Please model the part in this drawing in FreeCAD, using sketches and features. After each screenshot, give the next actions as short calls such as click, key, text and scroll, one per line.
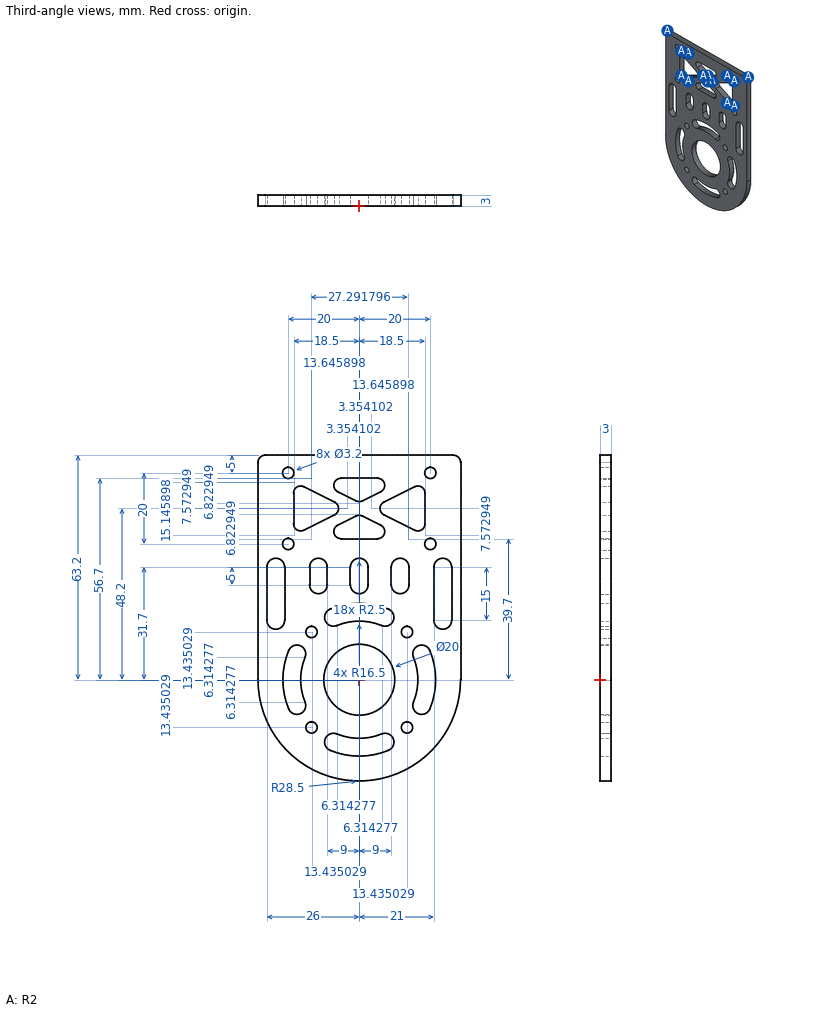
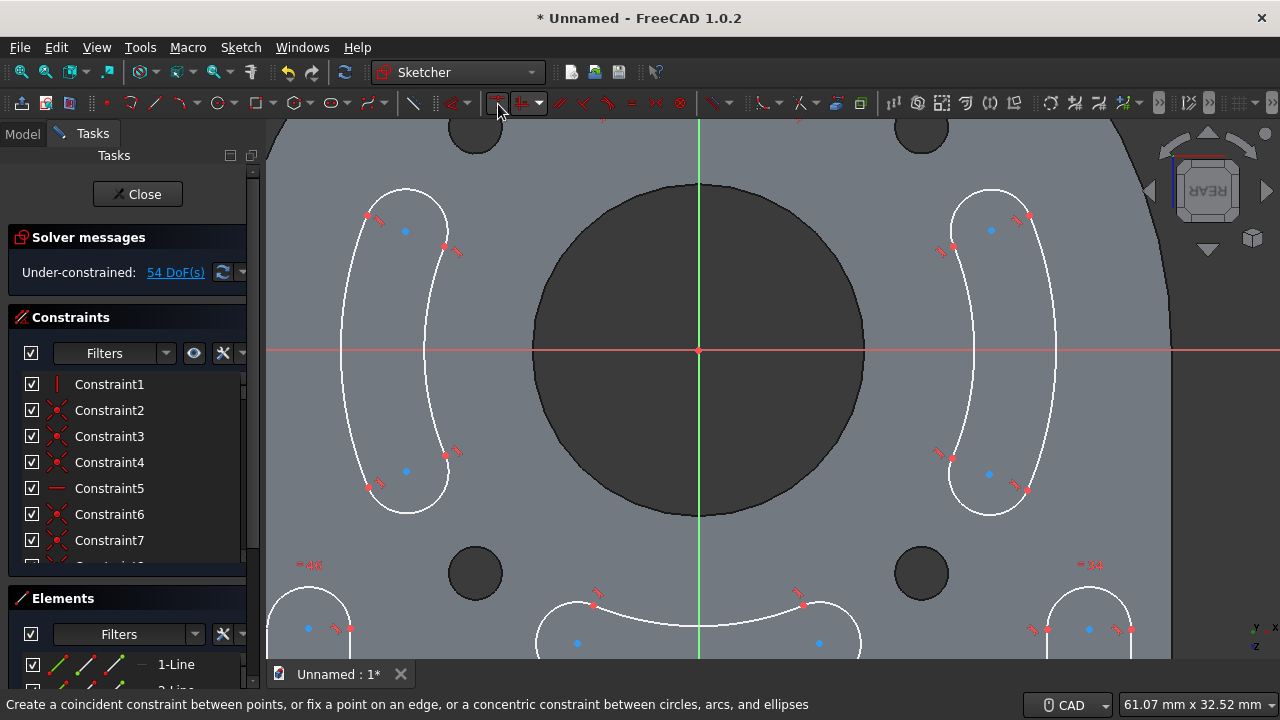
scroll(706, 306, down, 7)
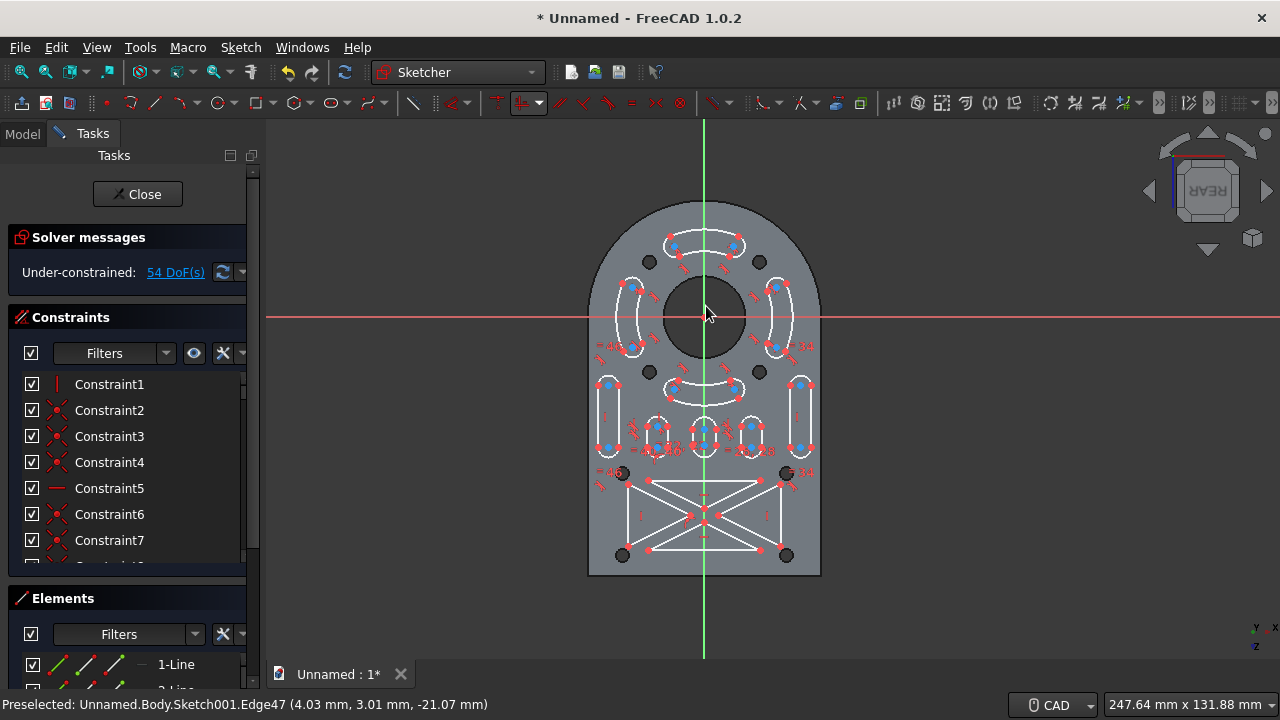
scroll(697, 455, up, 4)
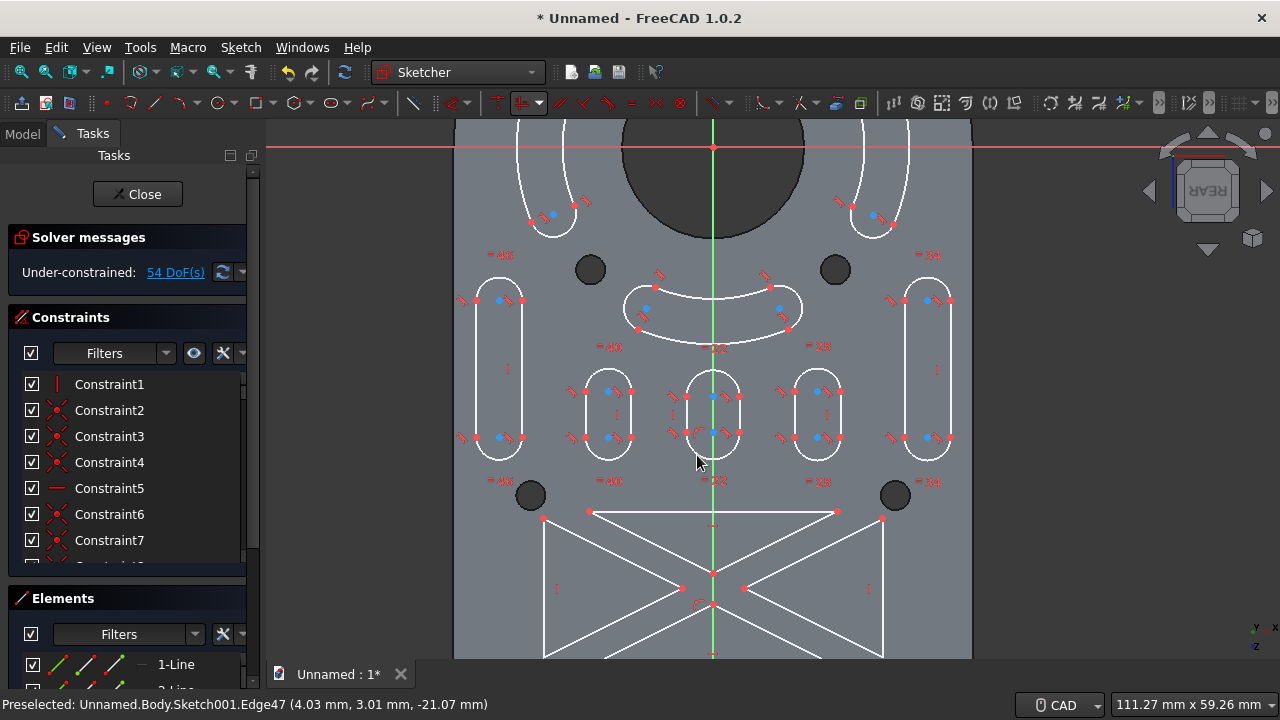
click(698, 454)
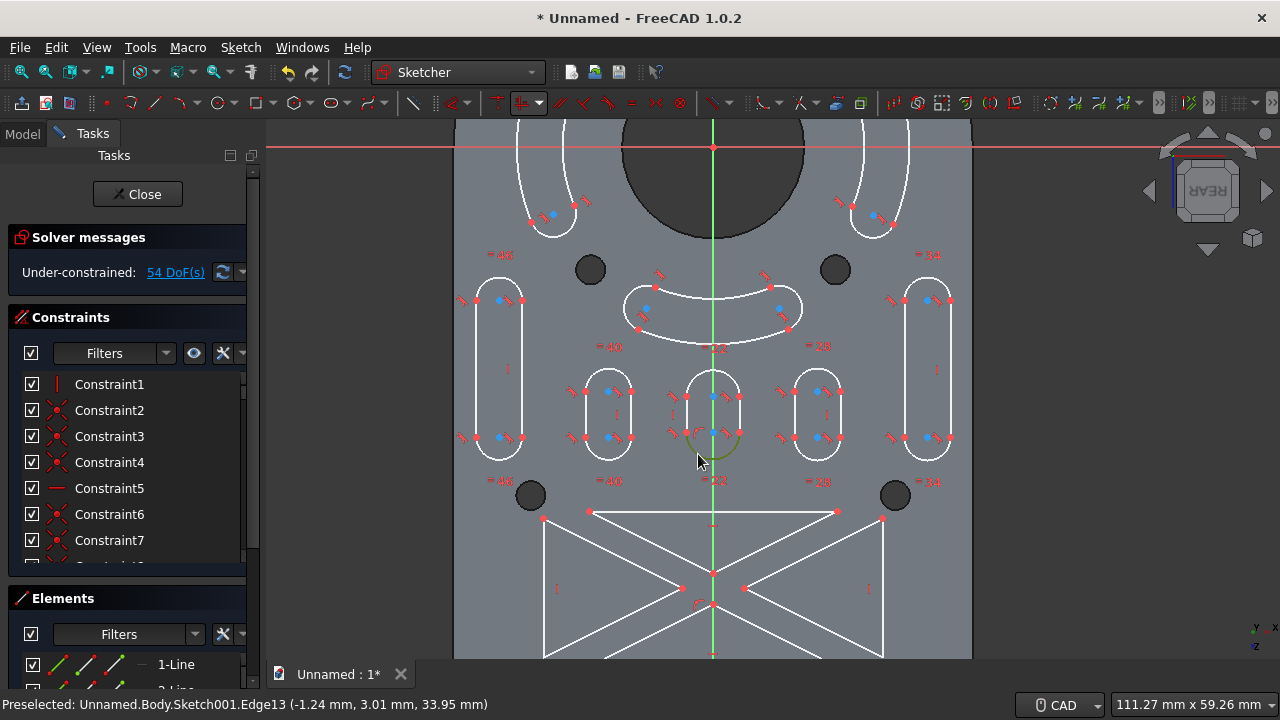
click(804, 456)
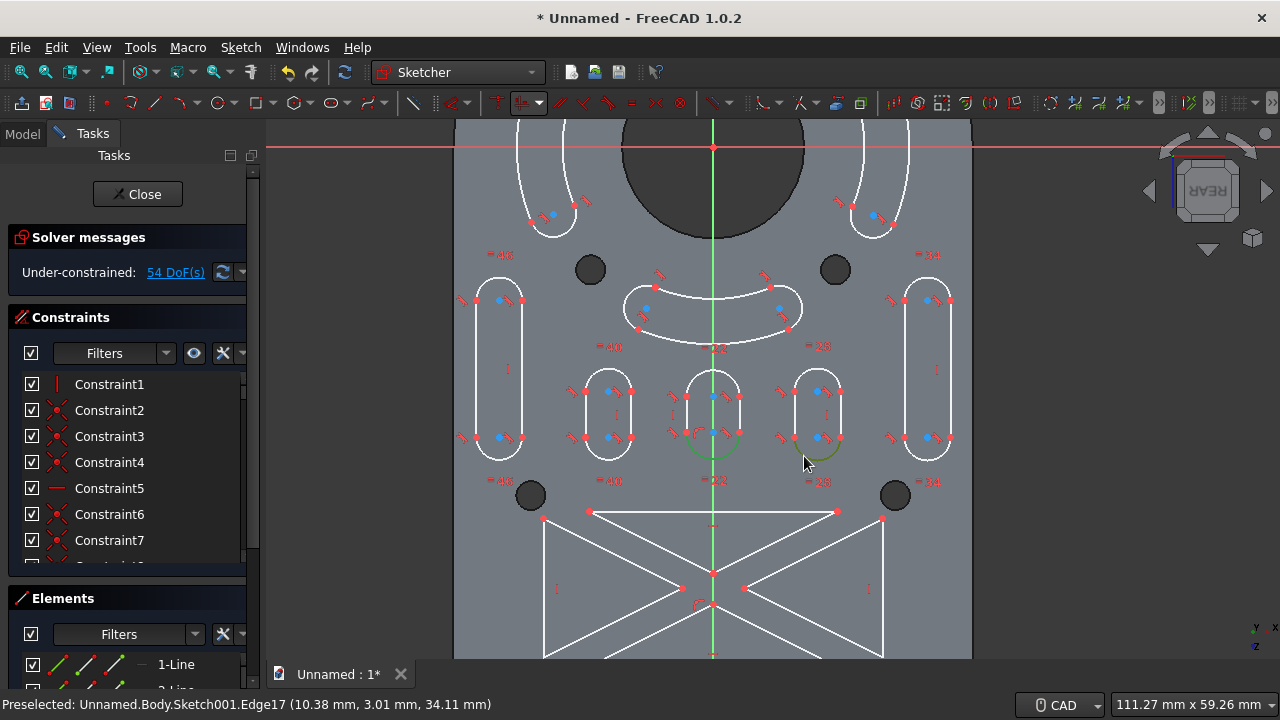
click(914, 456)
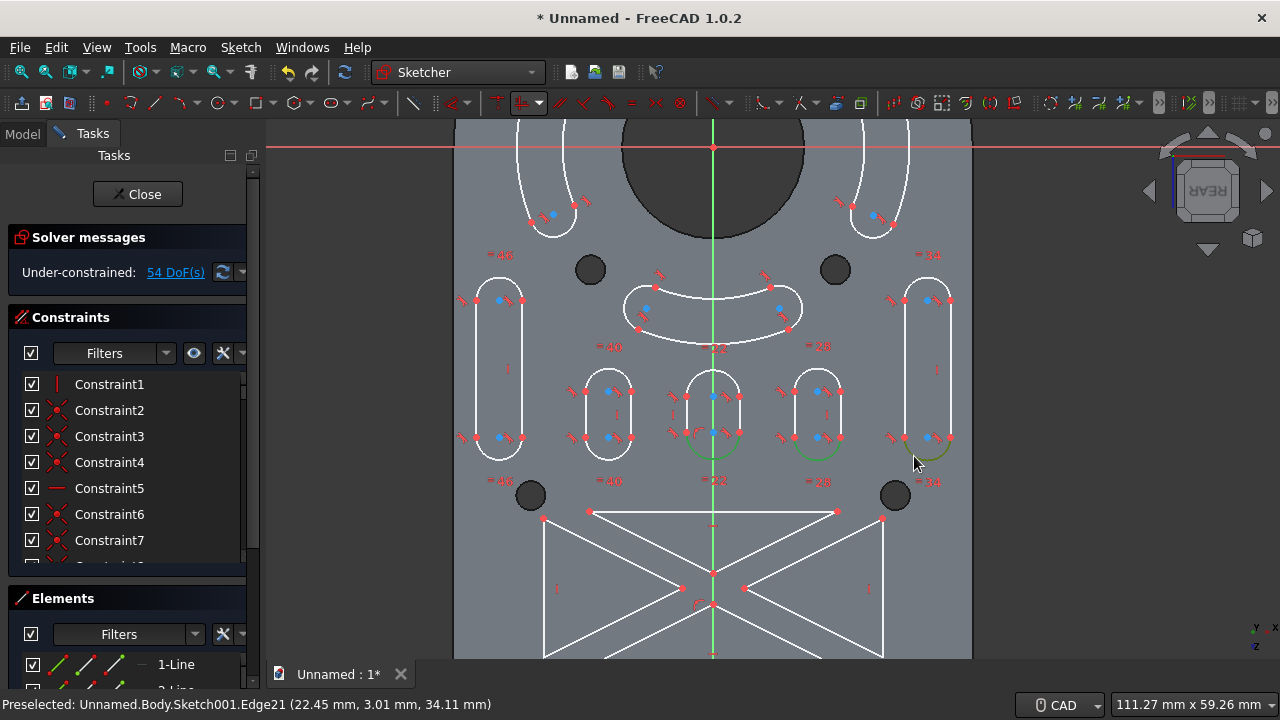
click(635, 289)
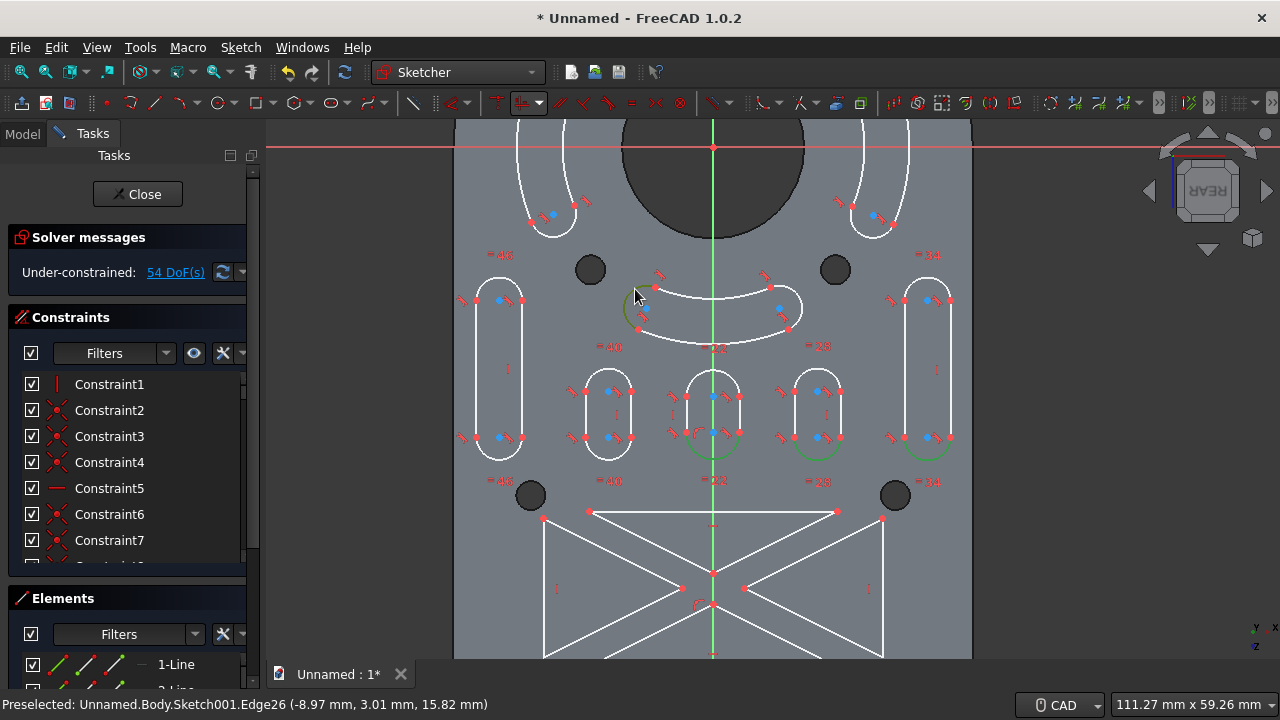
click(595, 455)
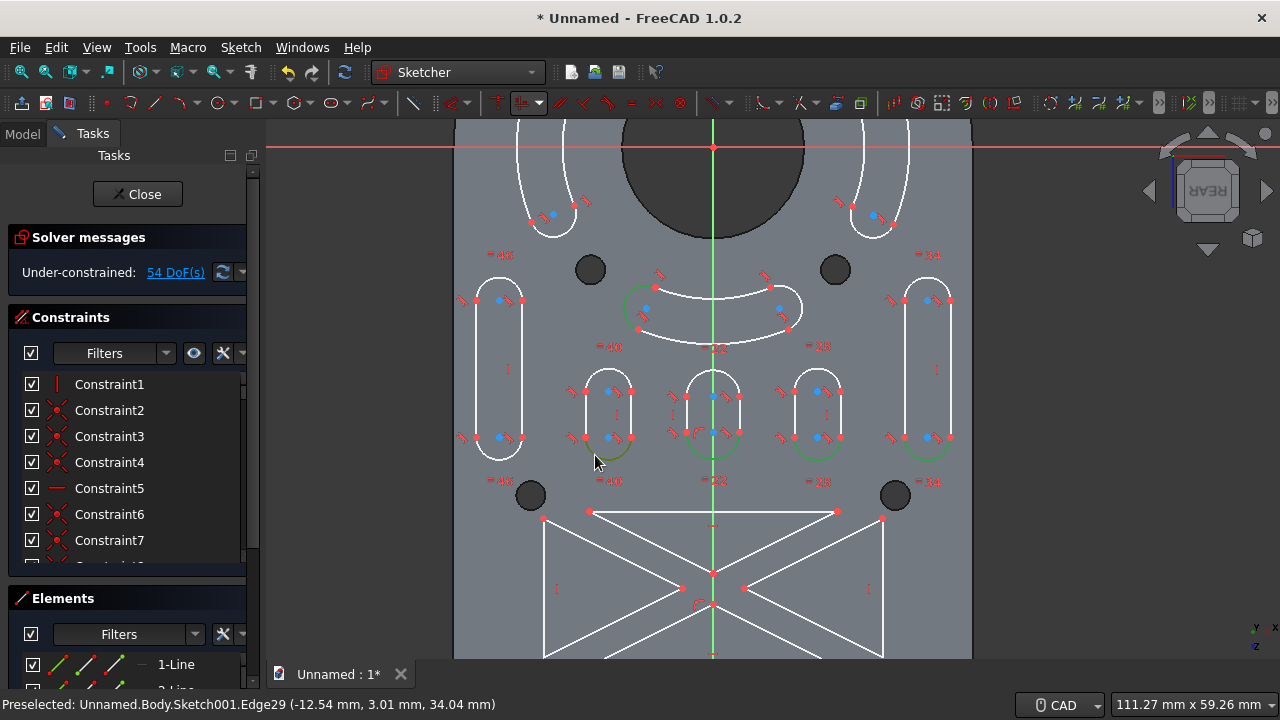
click(486, 455)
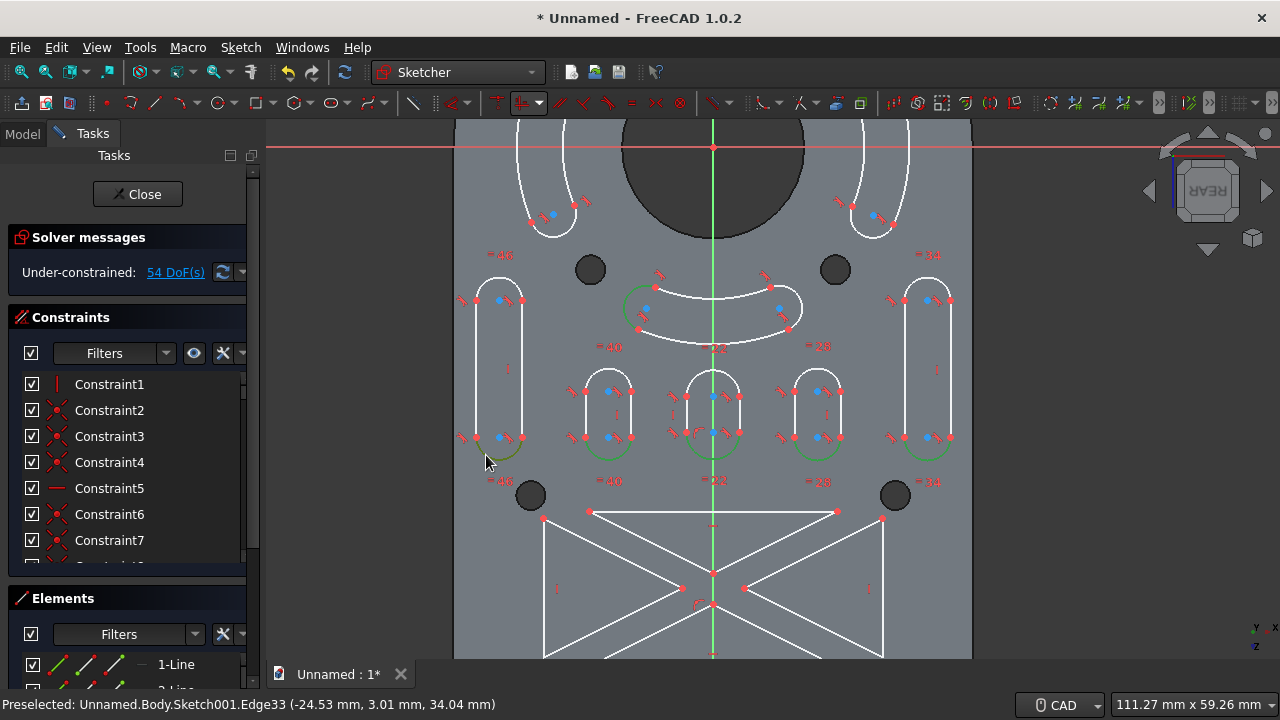
scroll(697, 455, down, 4)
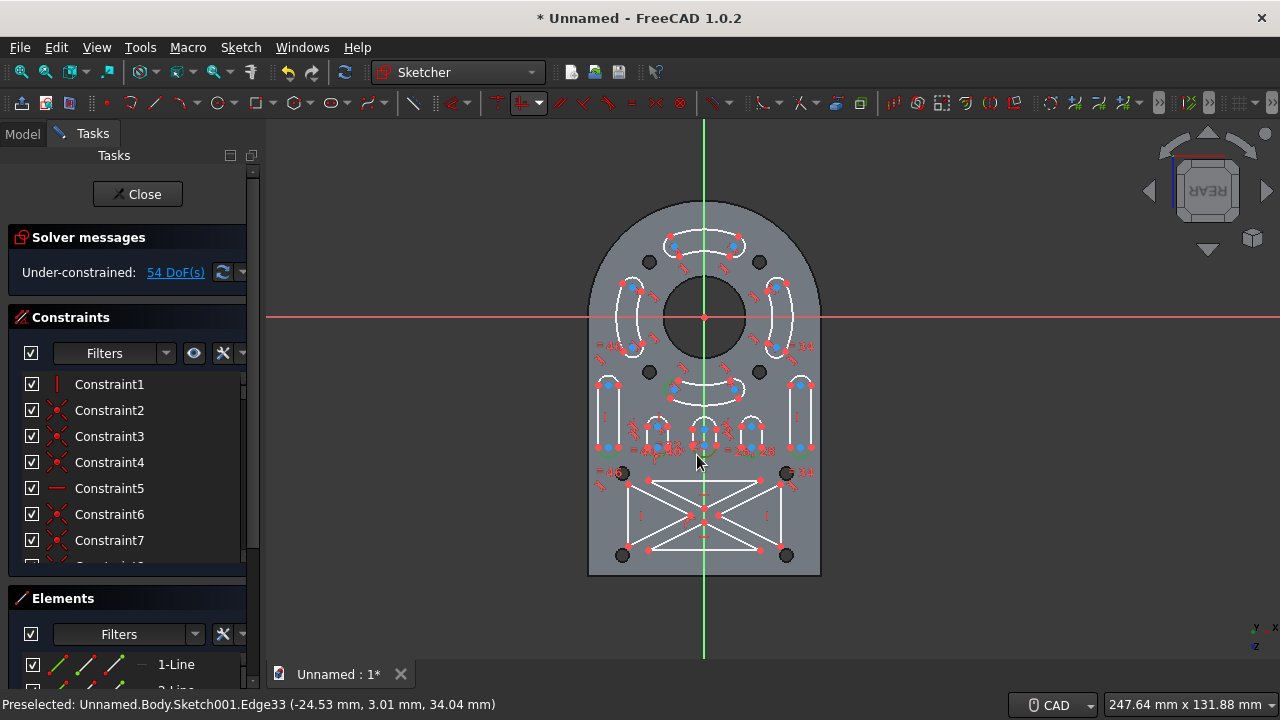
scroll(641, 282, up, 2)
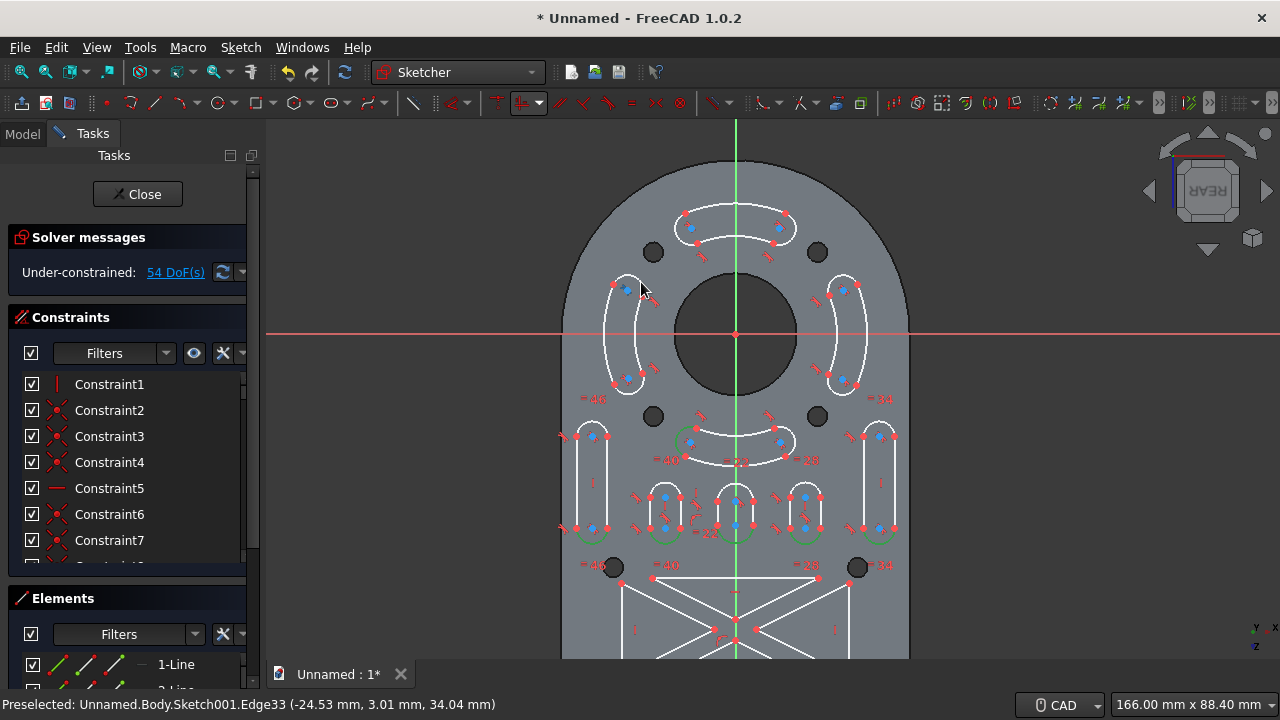
click(641, 282)